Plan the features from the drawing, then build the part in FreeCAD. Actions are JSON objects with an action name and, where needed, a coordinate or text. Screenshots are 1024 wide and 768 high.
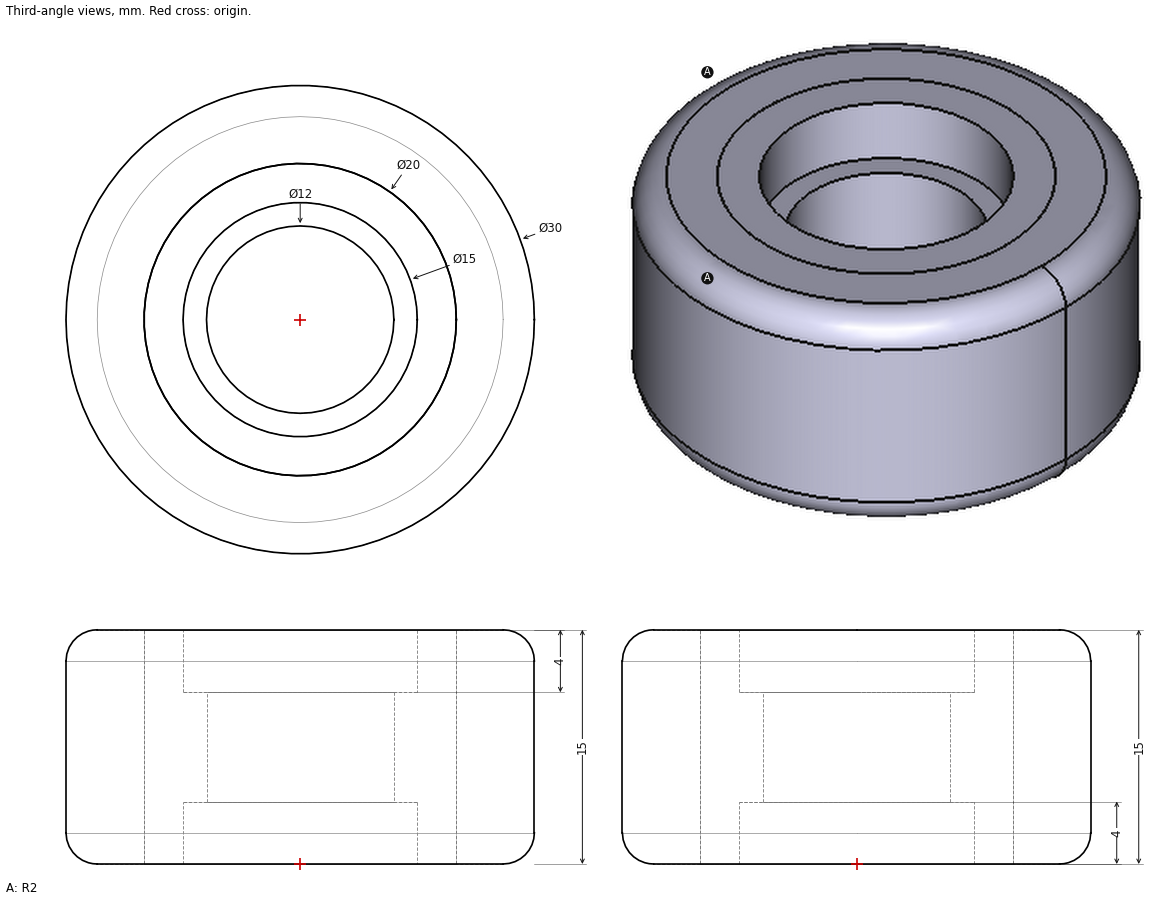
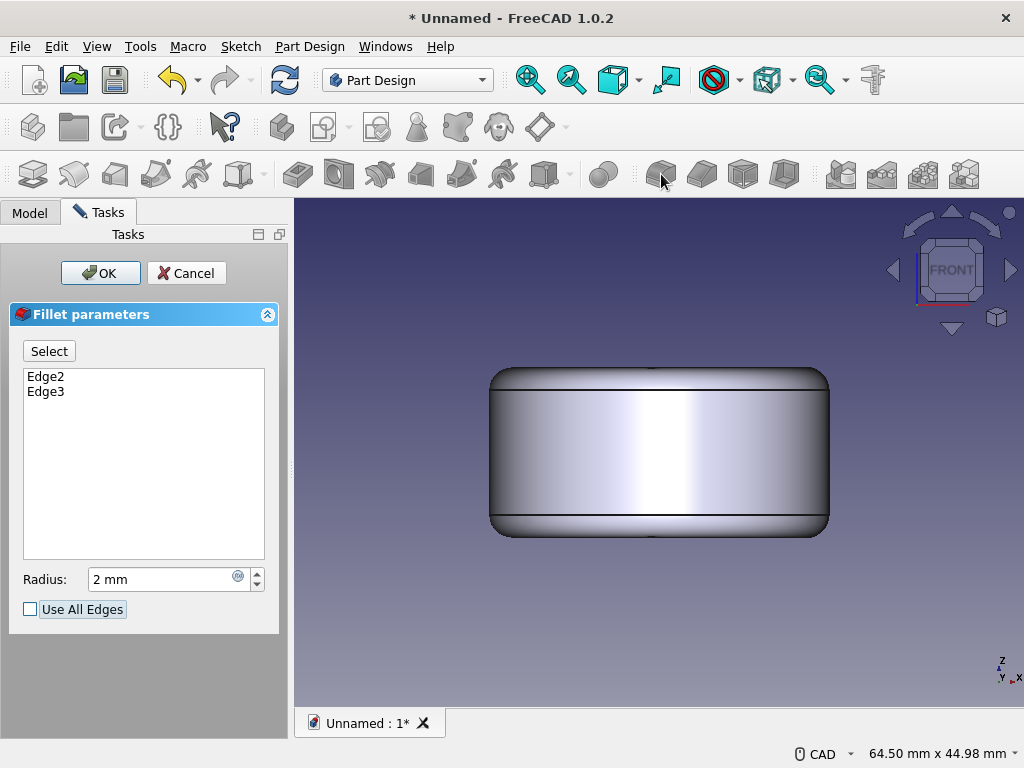
{"action": "left_click", "coordinate": [101, 273]}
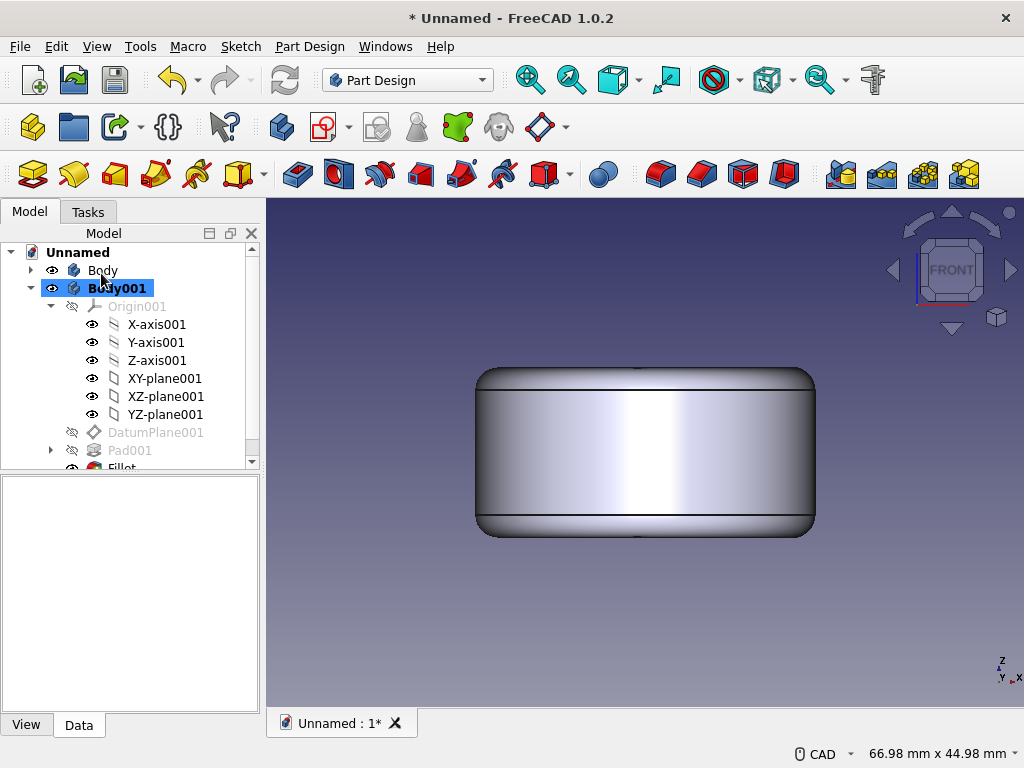
{"action": "key", "text": "0"}